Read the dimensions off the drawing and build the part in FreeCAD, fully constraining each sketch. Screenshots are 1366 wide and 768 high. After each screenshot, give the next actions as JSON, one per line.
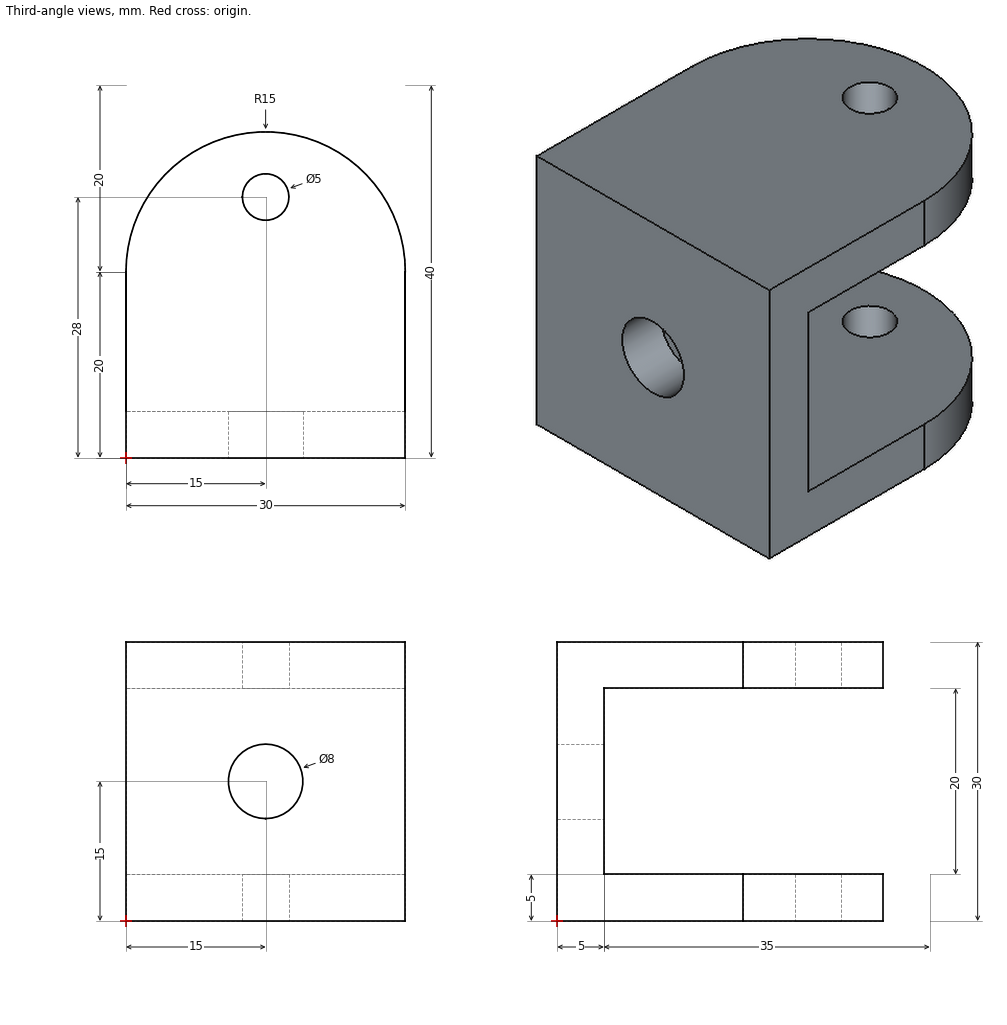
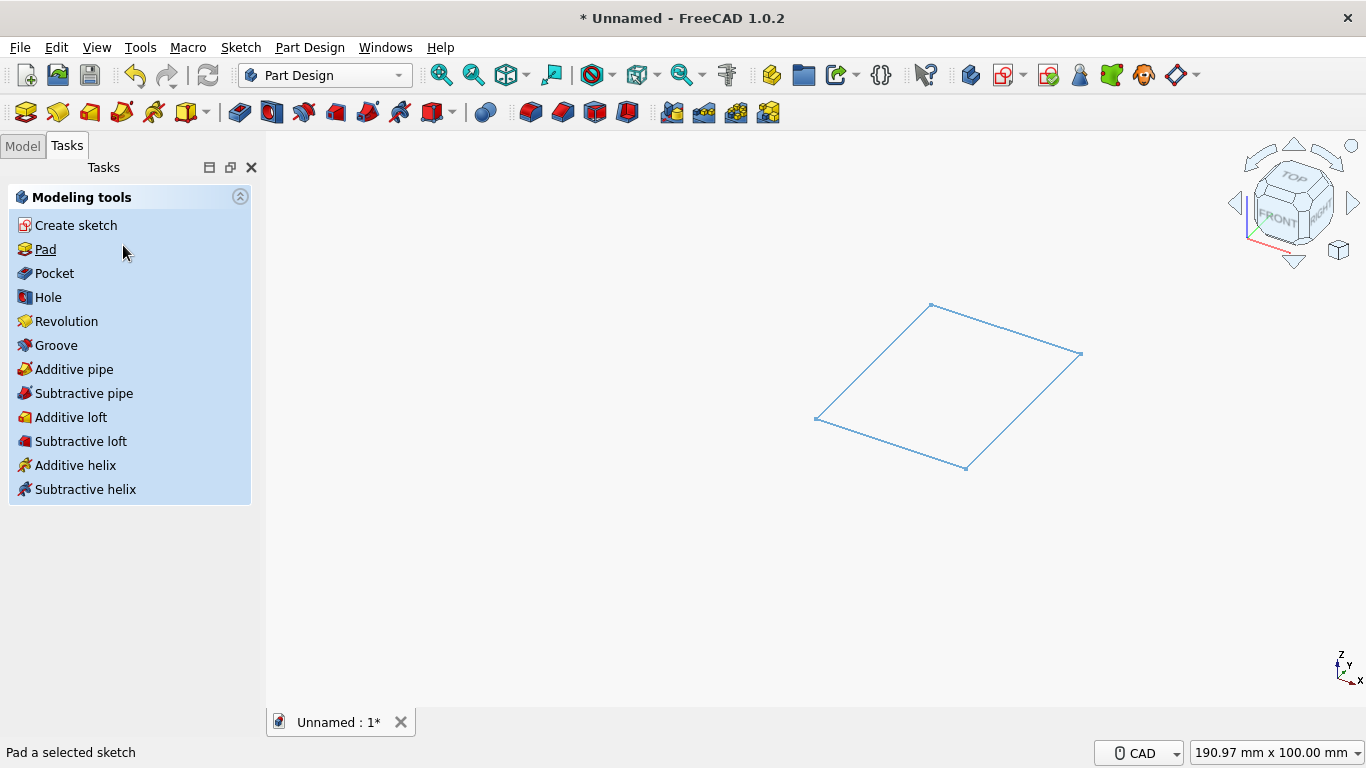
{"action": "left_click", "coordinate": [26, 112]}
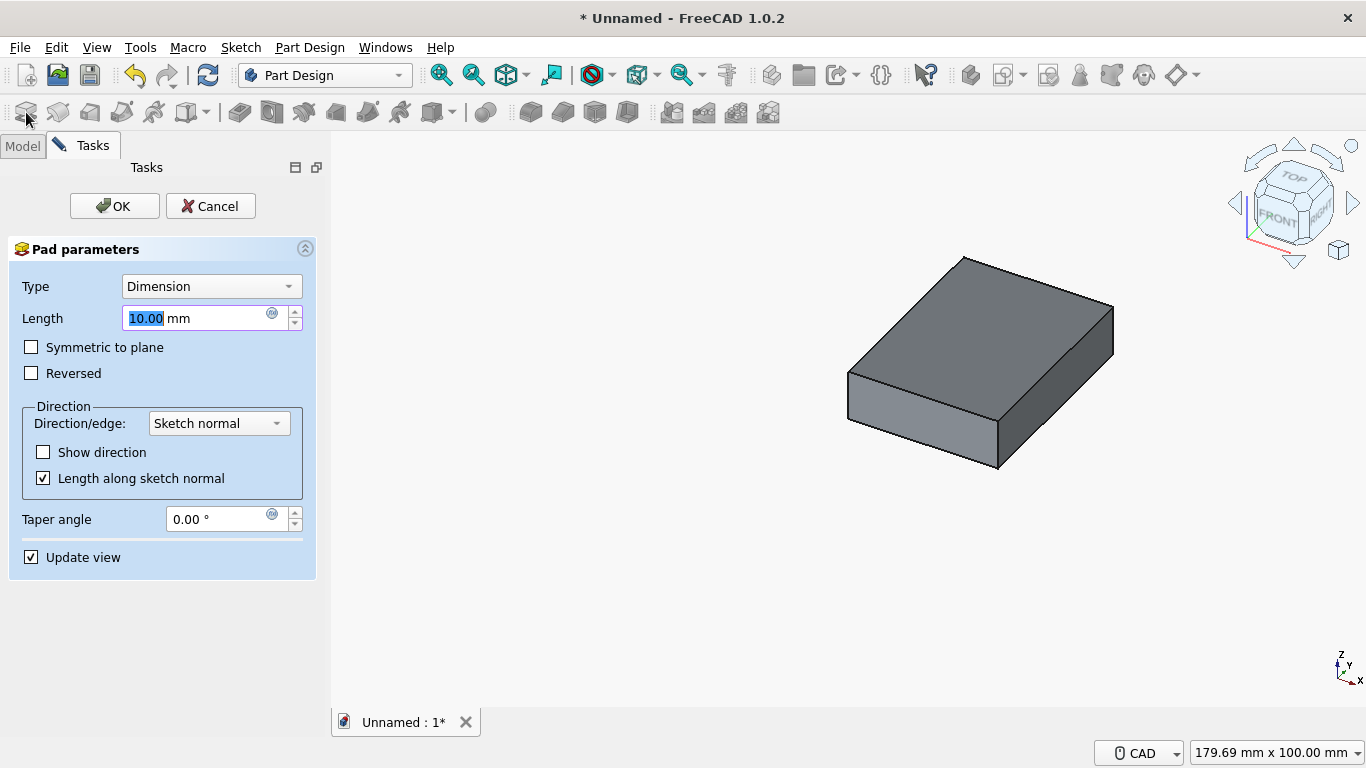
{"action": "type", "text": "30"}
{"action": "key", "text": "Tab"}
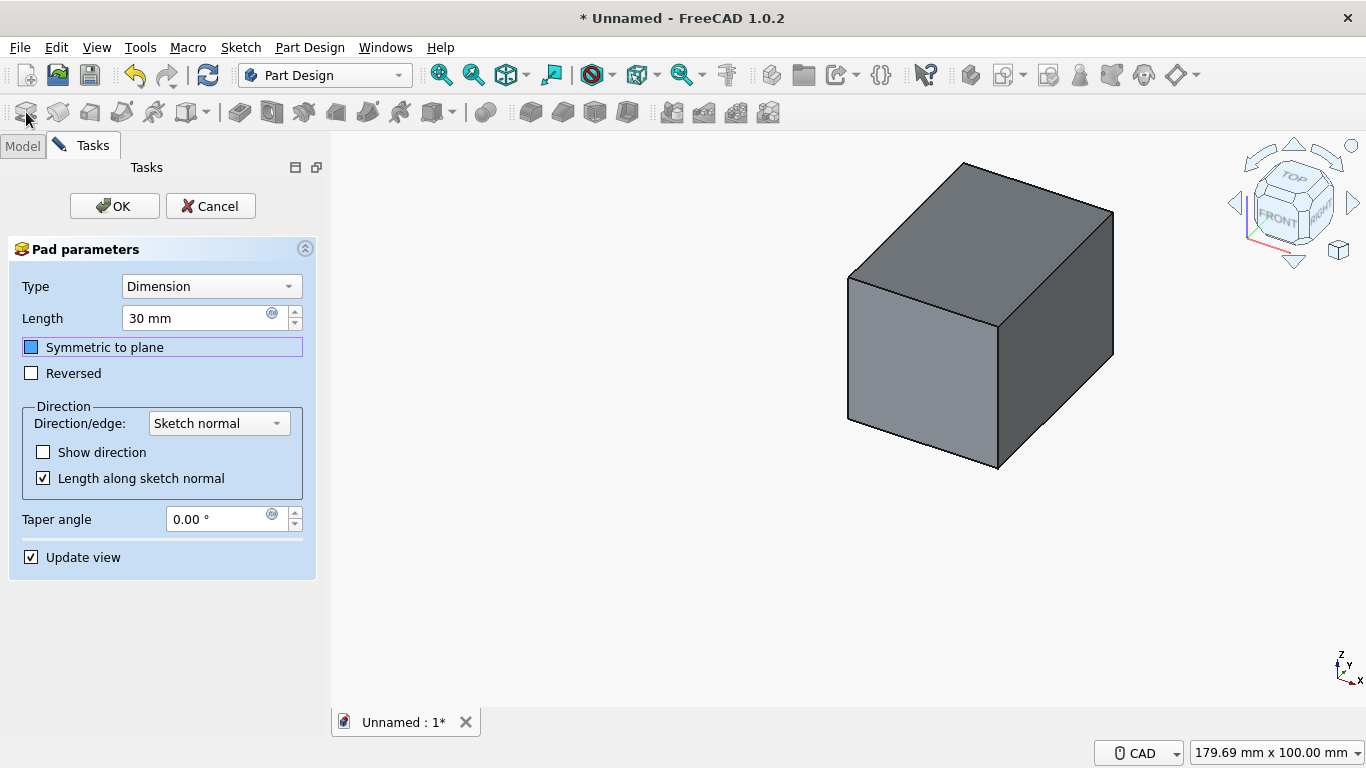
{"action": "left_click", "coordinate": [115, 206]}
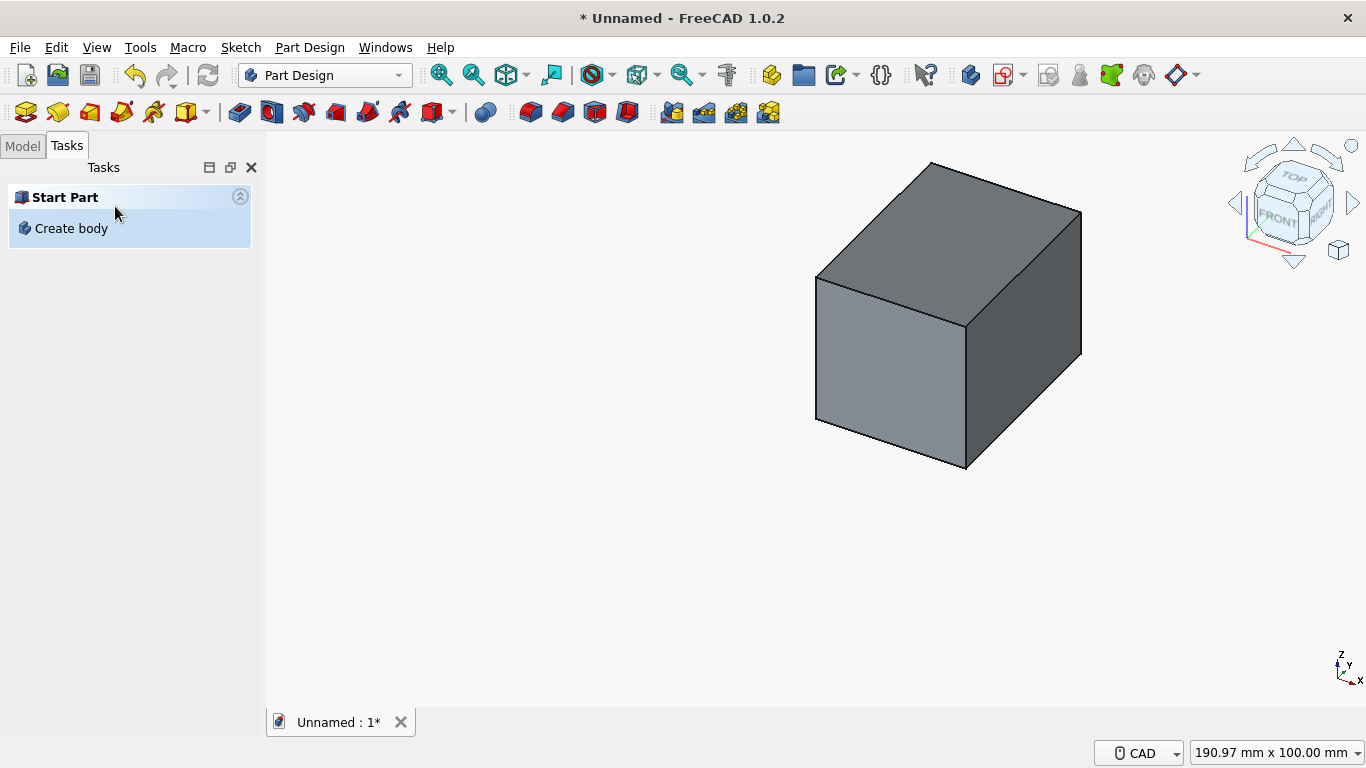
{"action": "left_click", "coordinate": [1023, 340]}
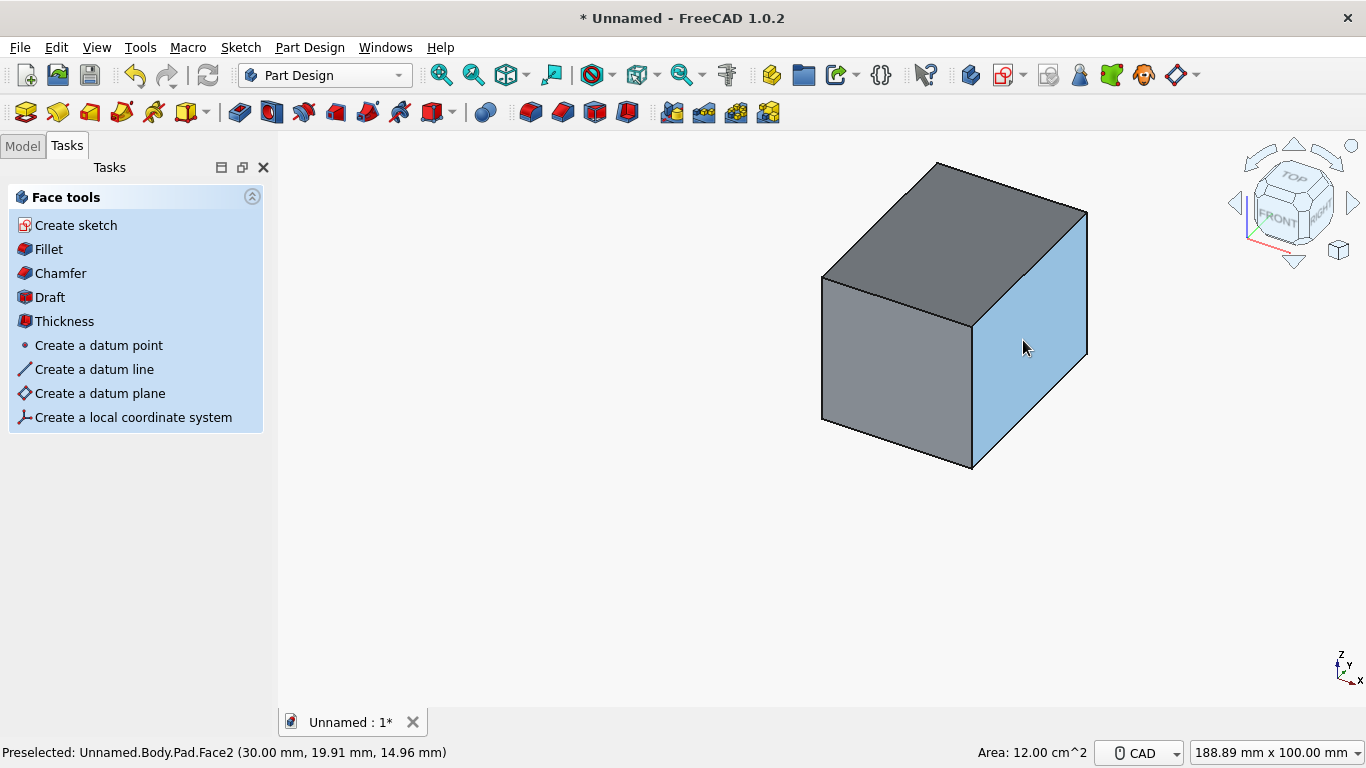
{"action": "left_click", "coordinate": [1004, 76]}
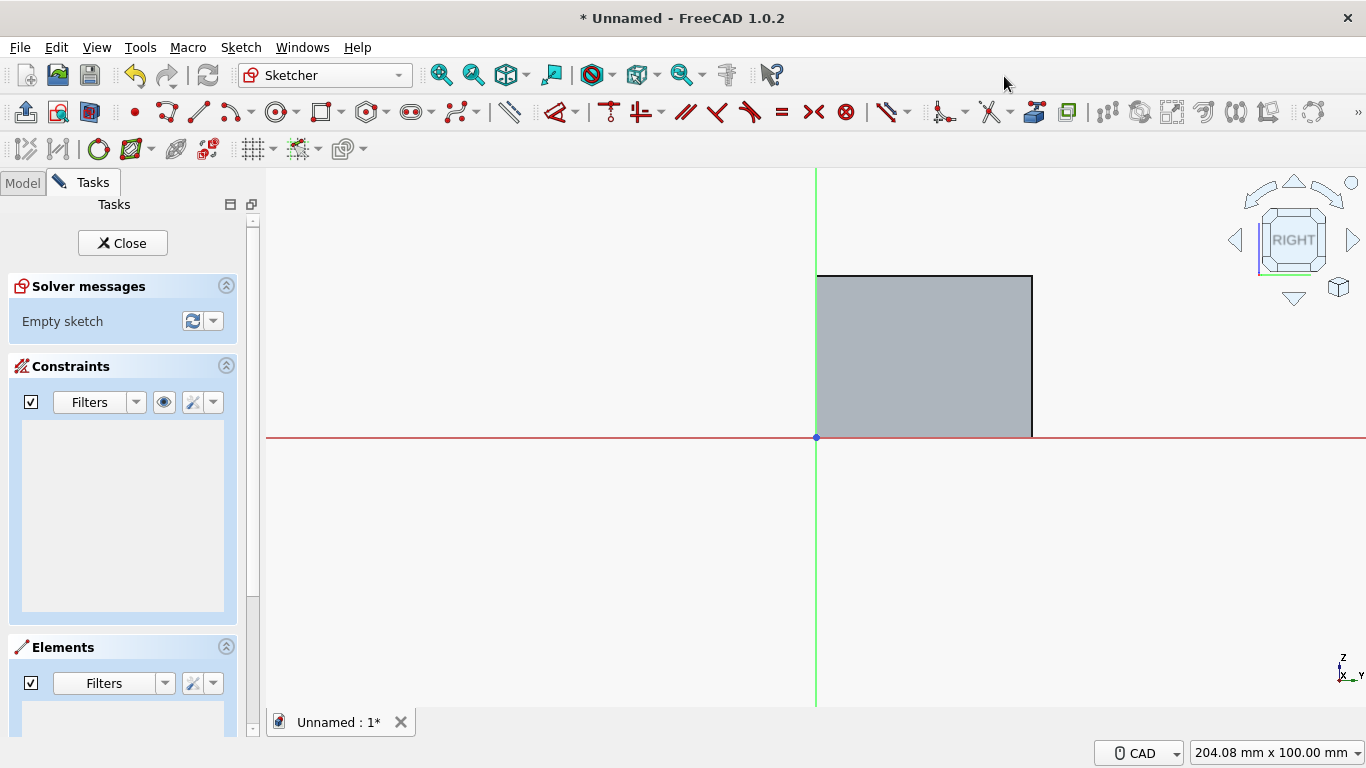
{"action": "scroll", "coordinate": [1026, 331], "scroll_direction": "up", "scroll_amount": 5}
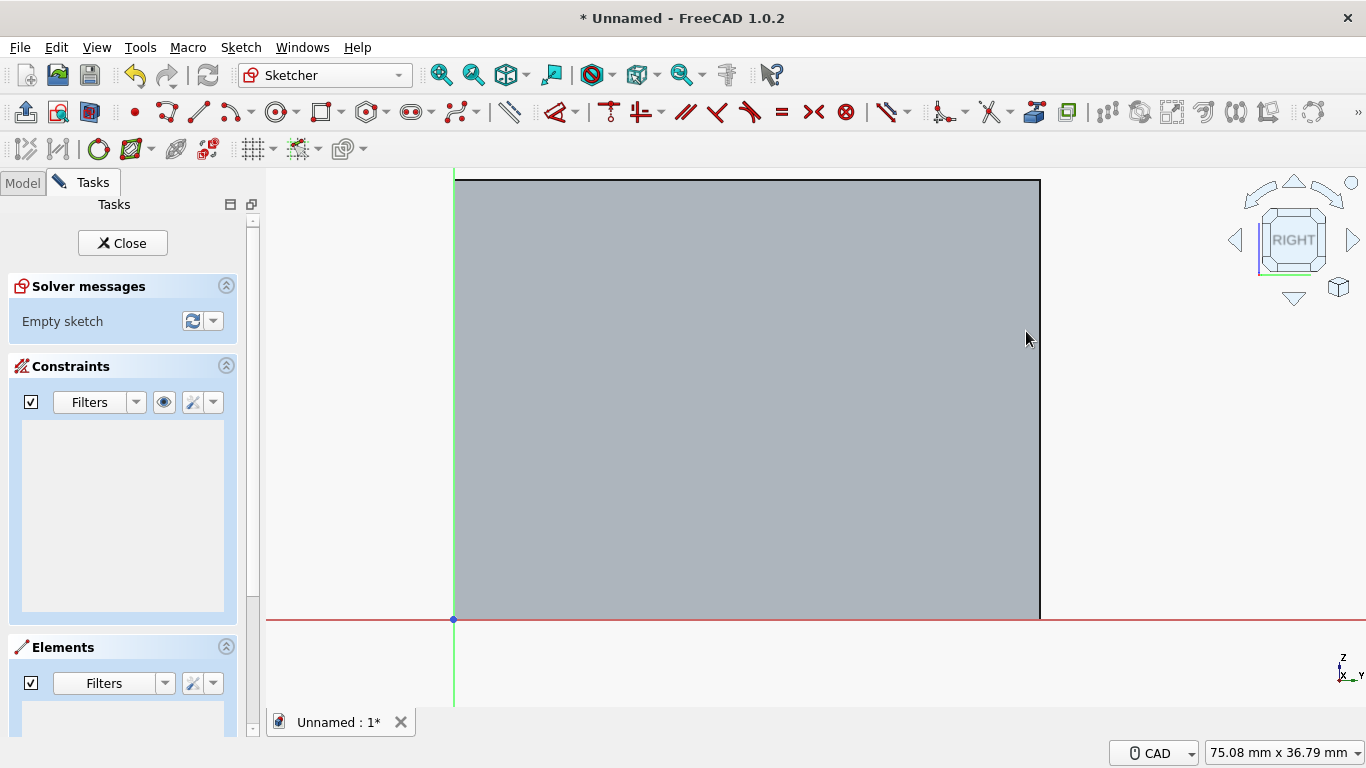
{"action": "left_click", "coordinate": [322, 112]}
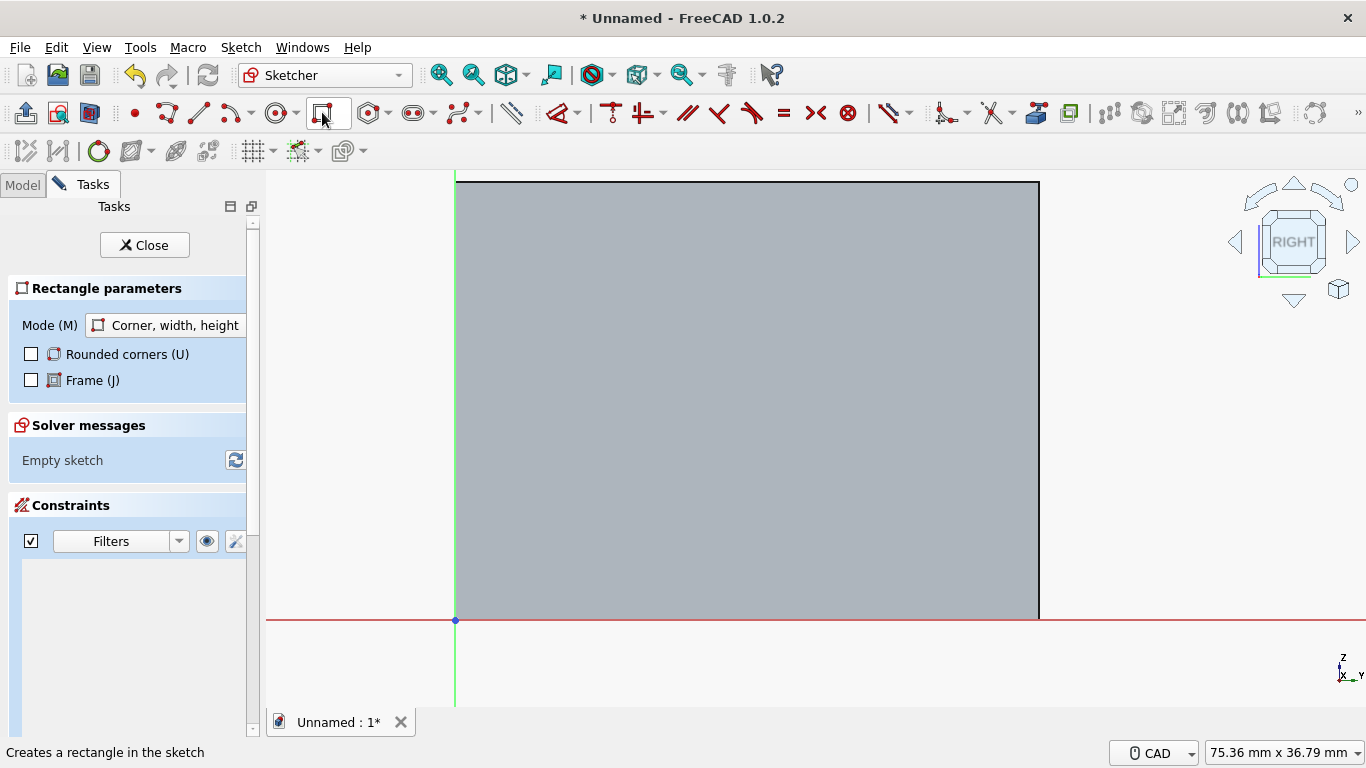
{"action": "left_click", "coordinate": [528, 255]}
{"action": "mouse_move", "coordinate": [1039, 547]}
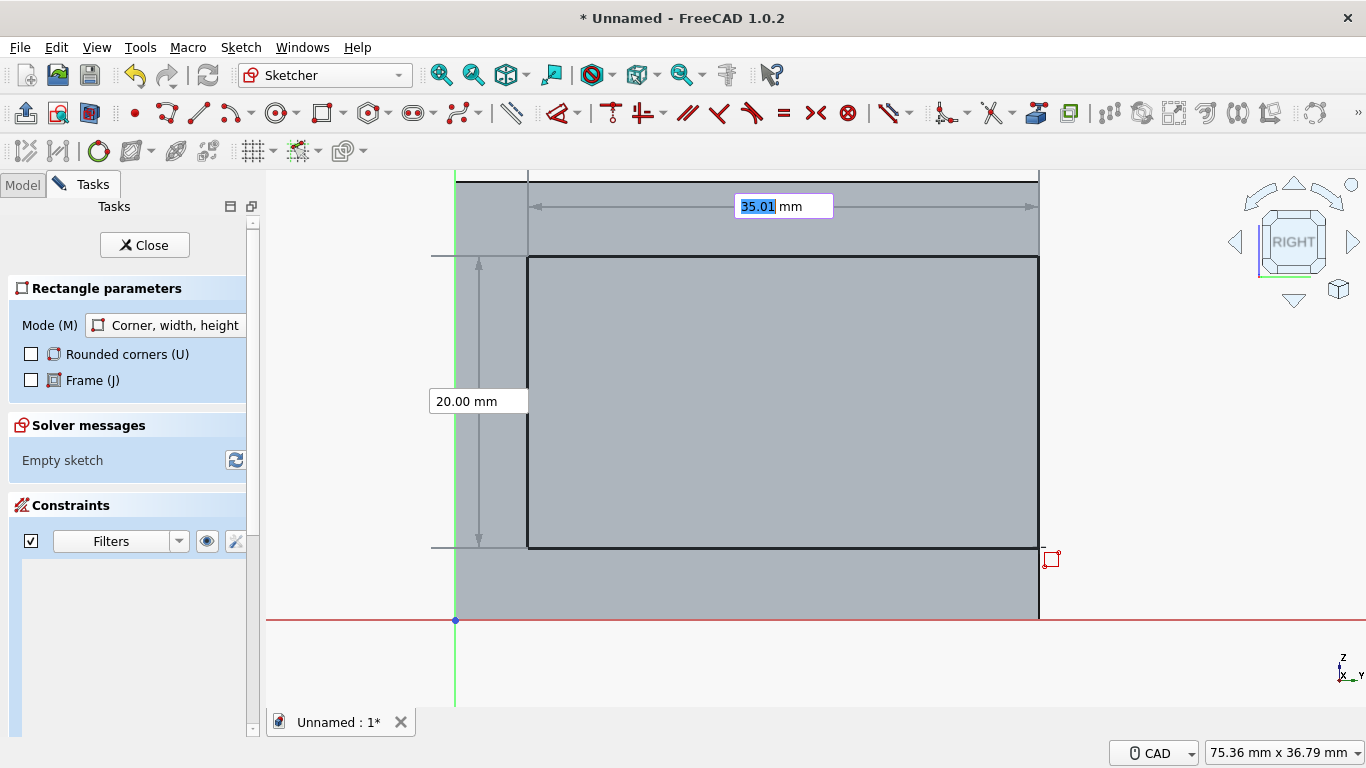
{"action": "type", "text": "35"}
{"action": "key", "text": "Tab"}
{"action": "type", "text": "20"}
{"action": "key", "text": "Return"}
{"action": "key", "text": "Escape"}